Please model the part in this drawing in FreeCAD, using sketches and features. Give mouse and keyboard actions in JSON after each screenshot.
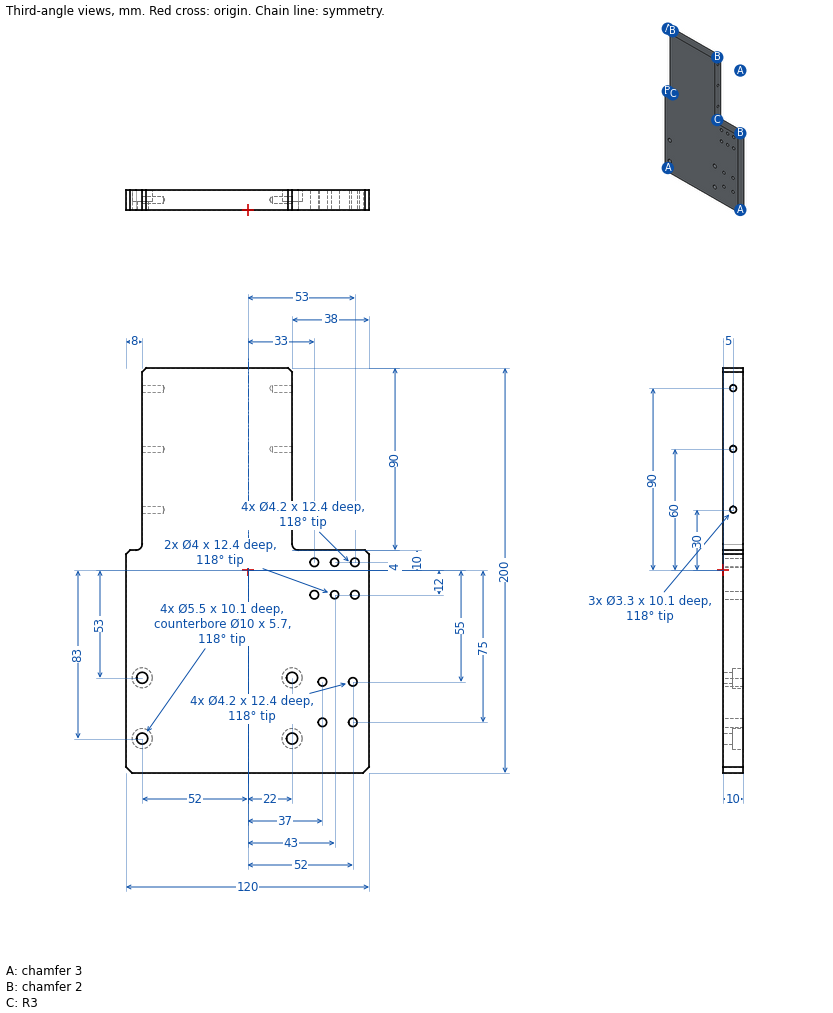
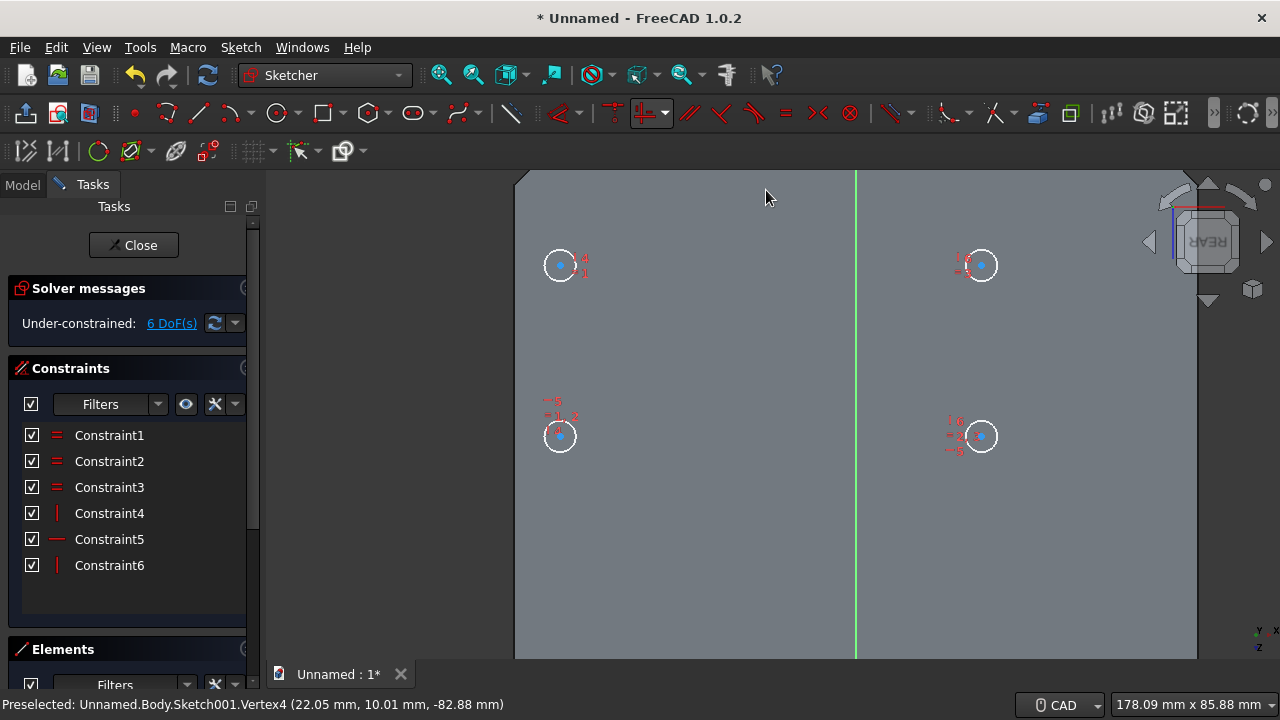
{"action": "left_click", "coordinate": [560, 266]}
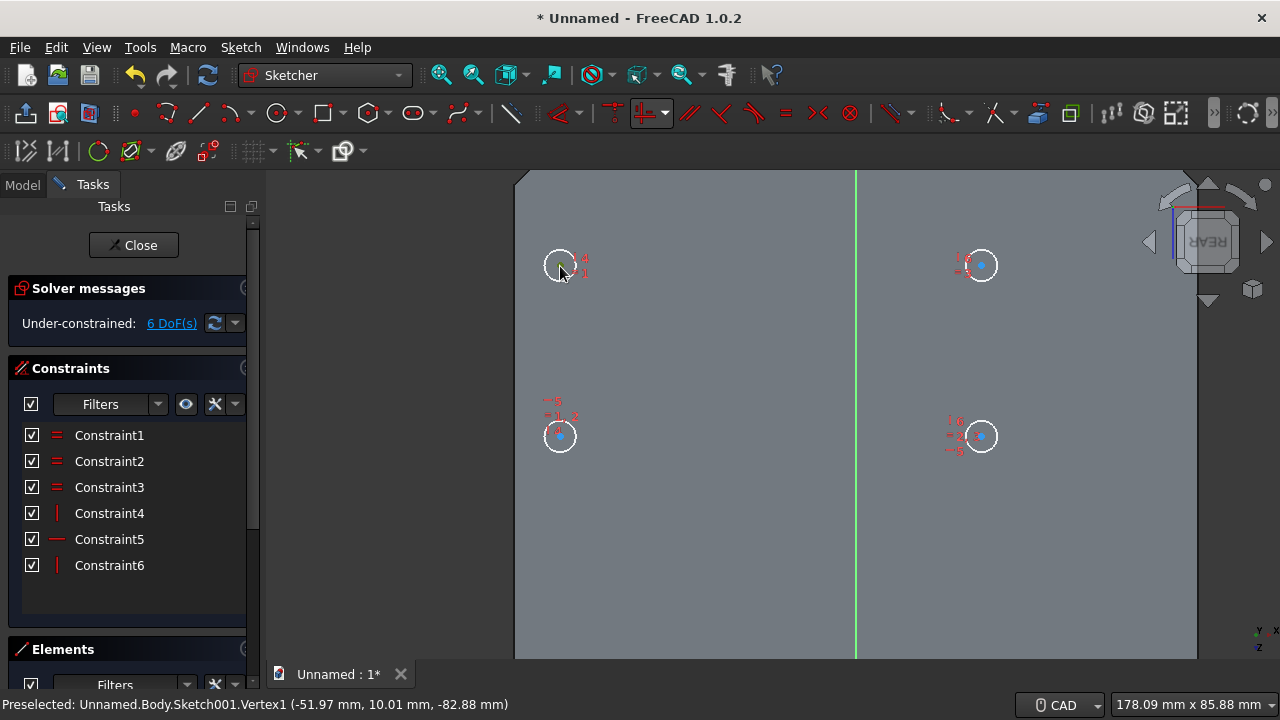
{"action": "left_click", "coordinate": [982, 266]}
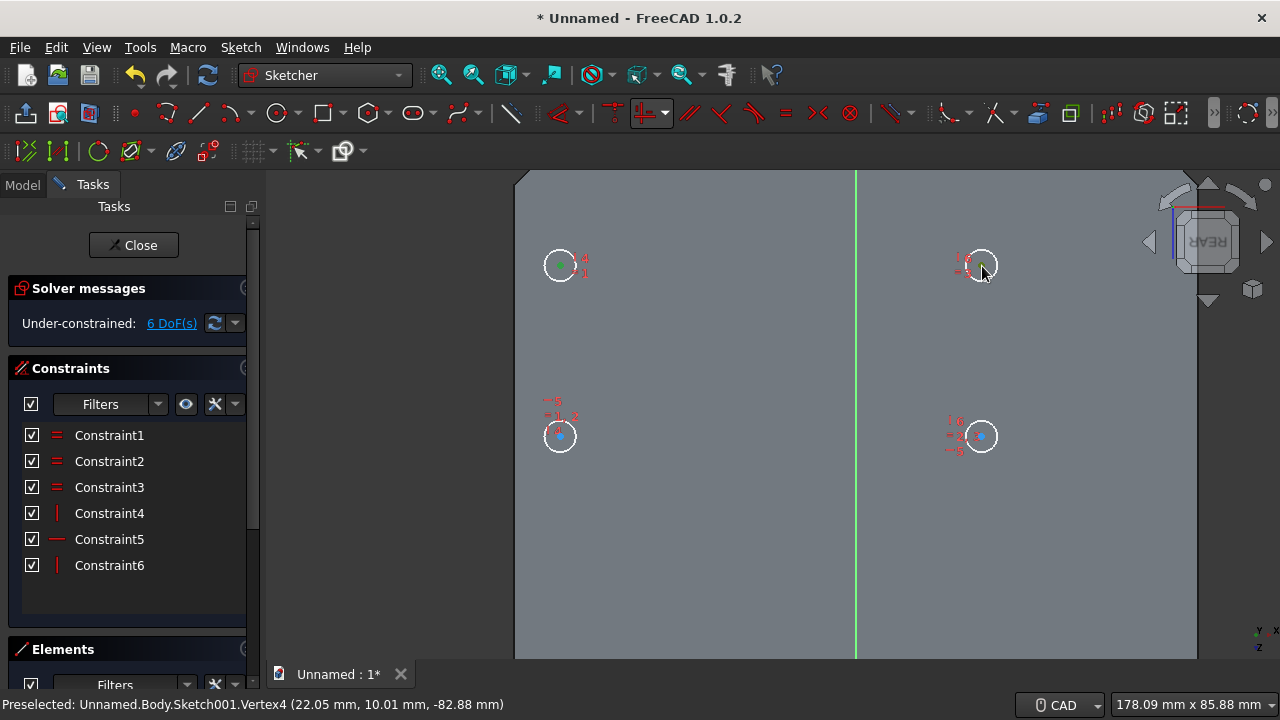
{"action": "key", "text": "h"}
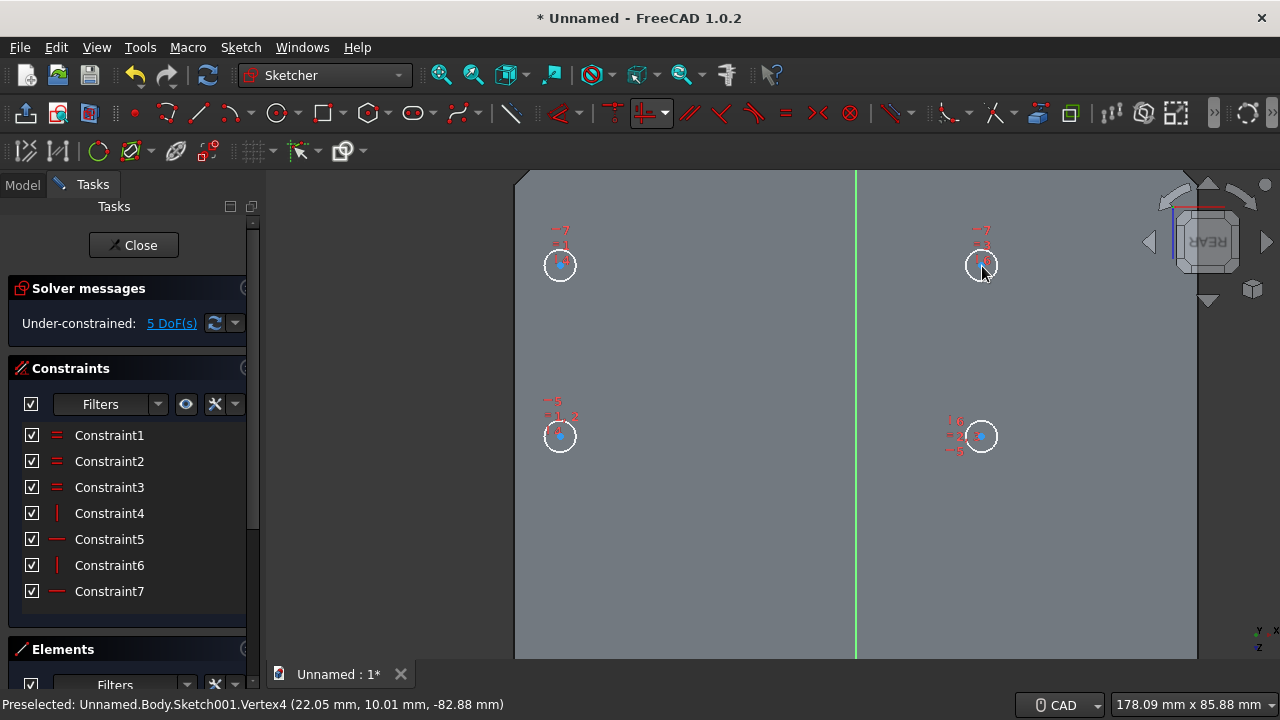
{"action": "left_click", "coordinate": [558, 114]}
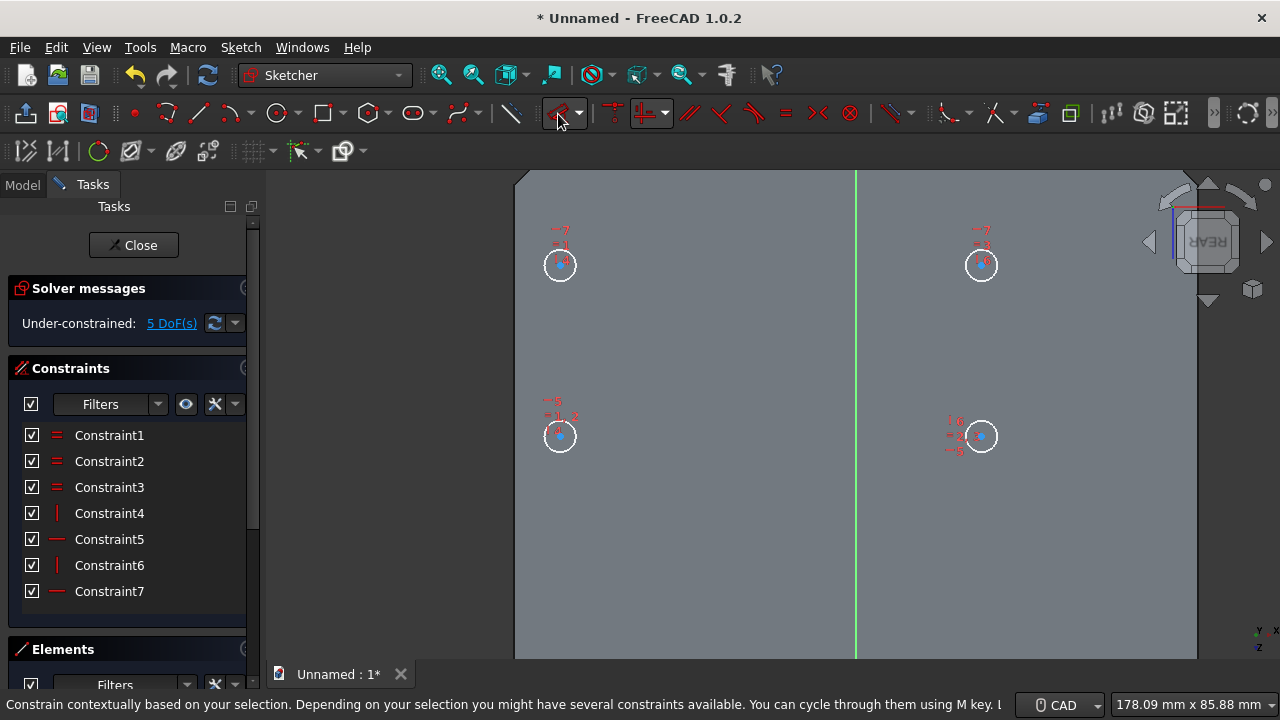
{"action": "scroll", "coordinate": [571, 254], "scroll_direction": "up", "scroll_amount": 2}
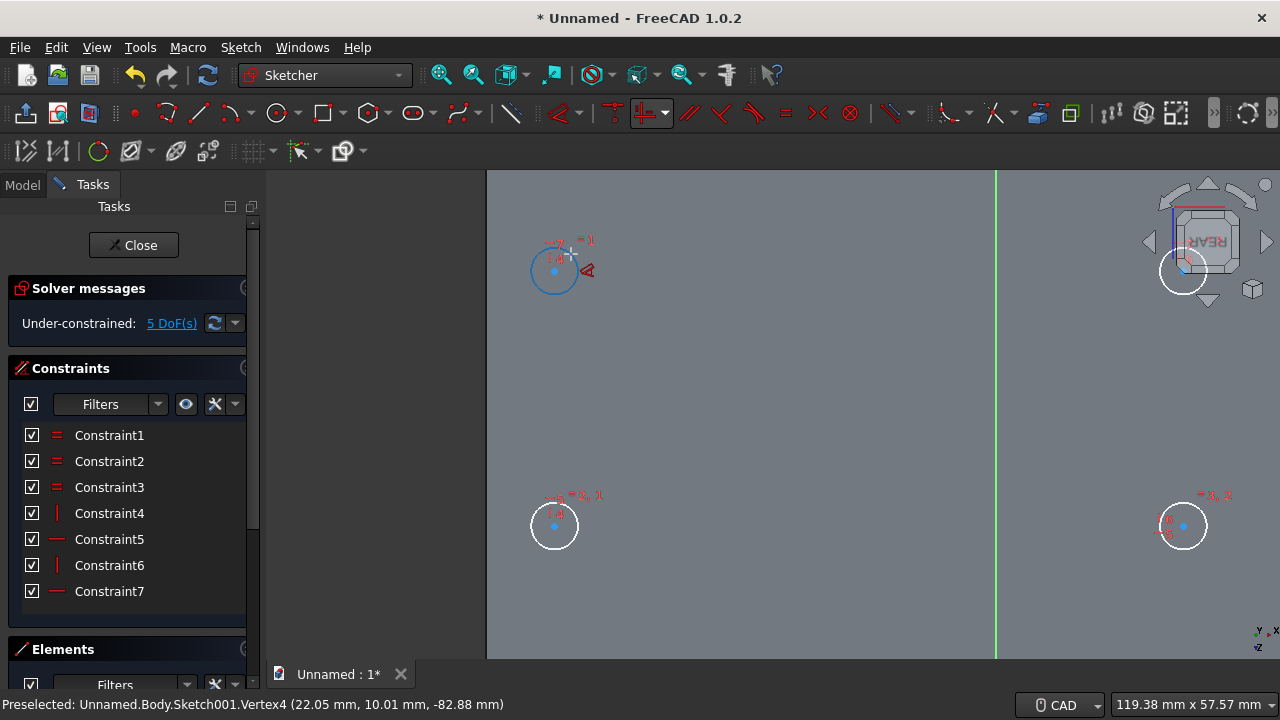
{"action": "left_click", "coordinate": [571, 255]}
{"action": "left_click", "coordinate": [594, 233]}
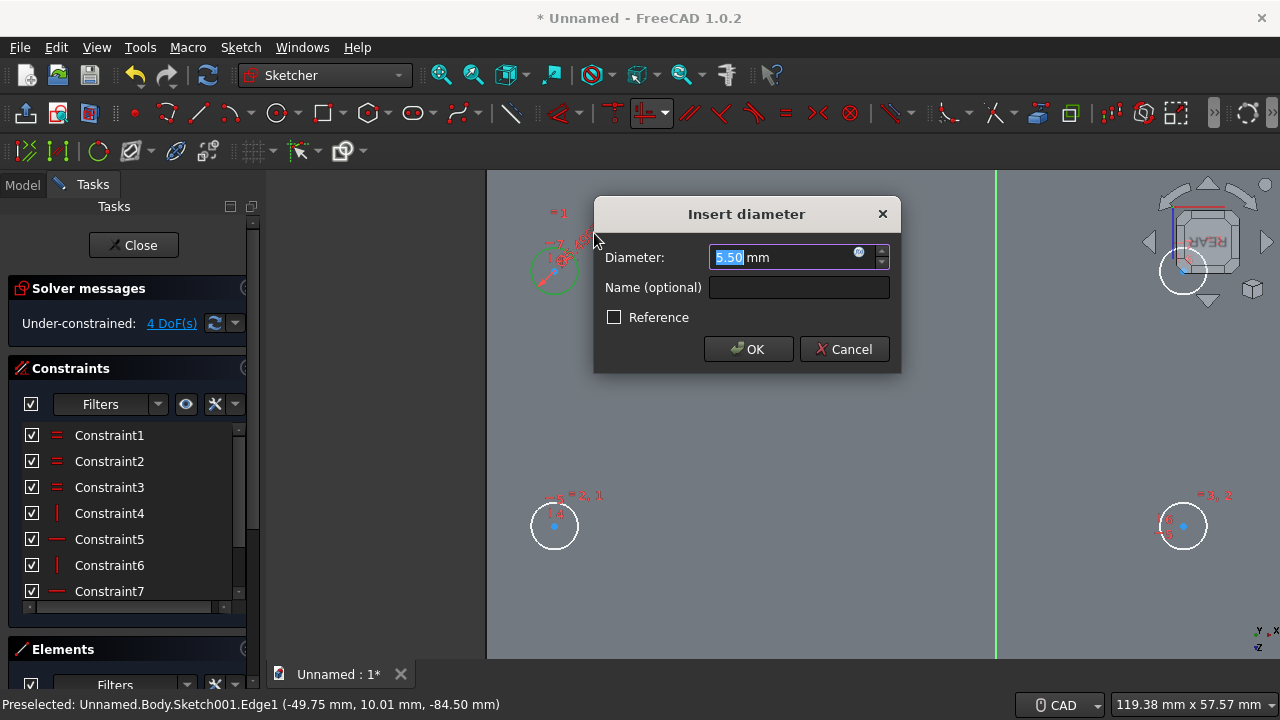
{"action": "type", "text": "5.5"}
{"action": "key", "text": "Return"}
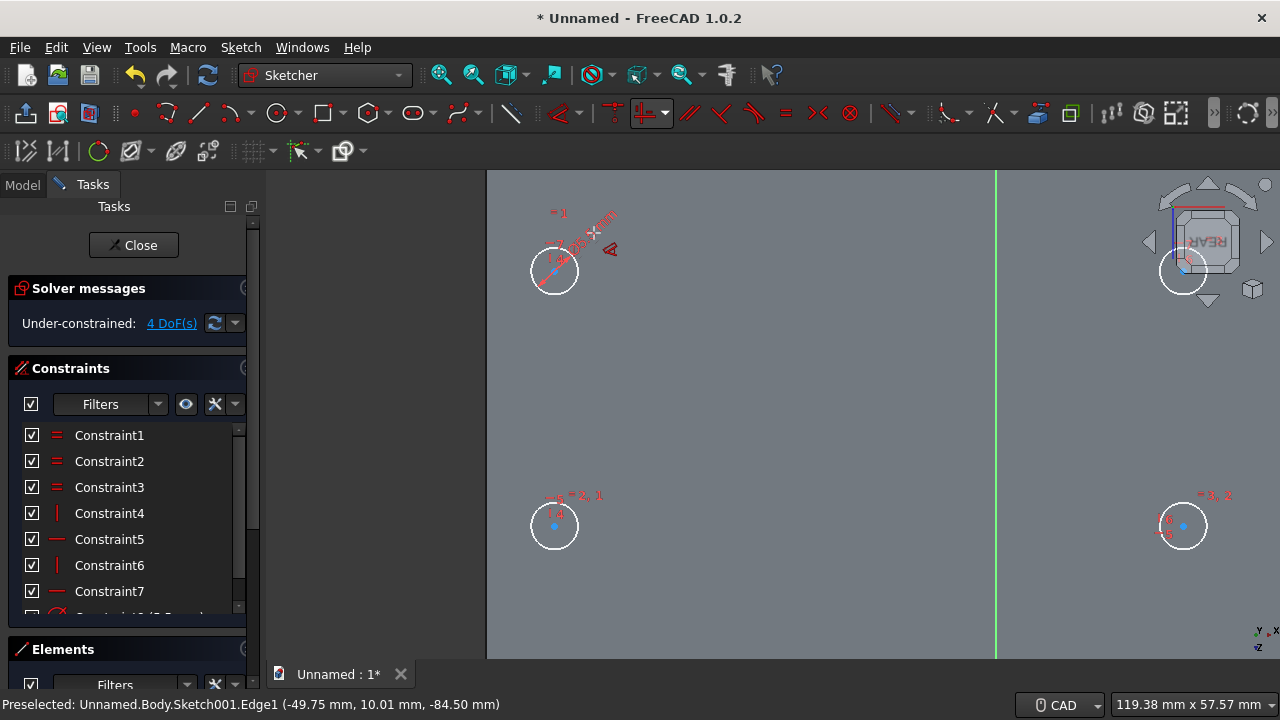
{"action": "left_click", "coordinate": [555, 271]}
{"action": "left_click", "coordinate": [775, 237]}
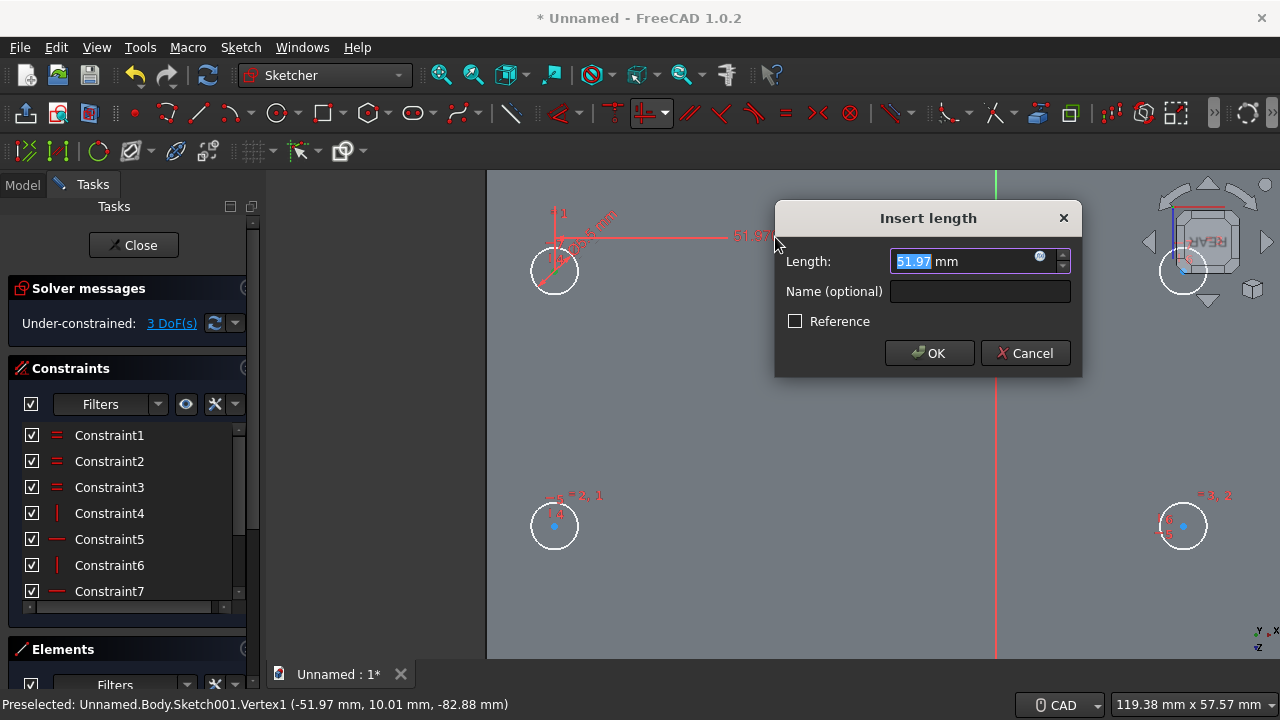
{"action": "type", "text": "52"}
{"action": "key", "text": "Return"}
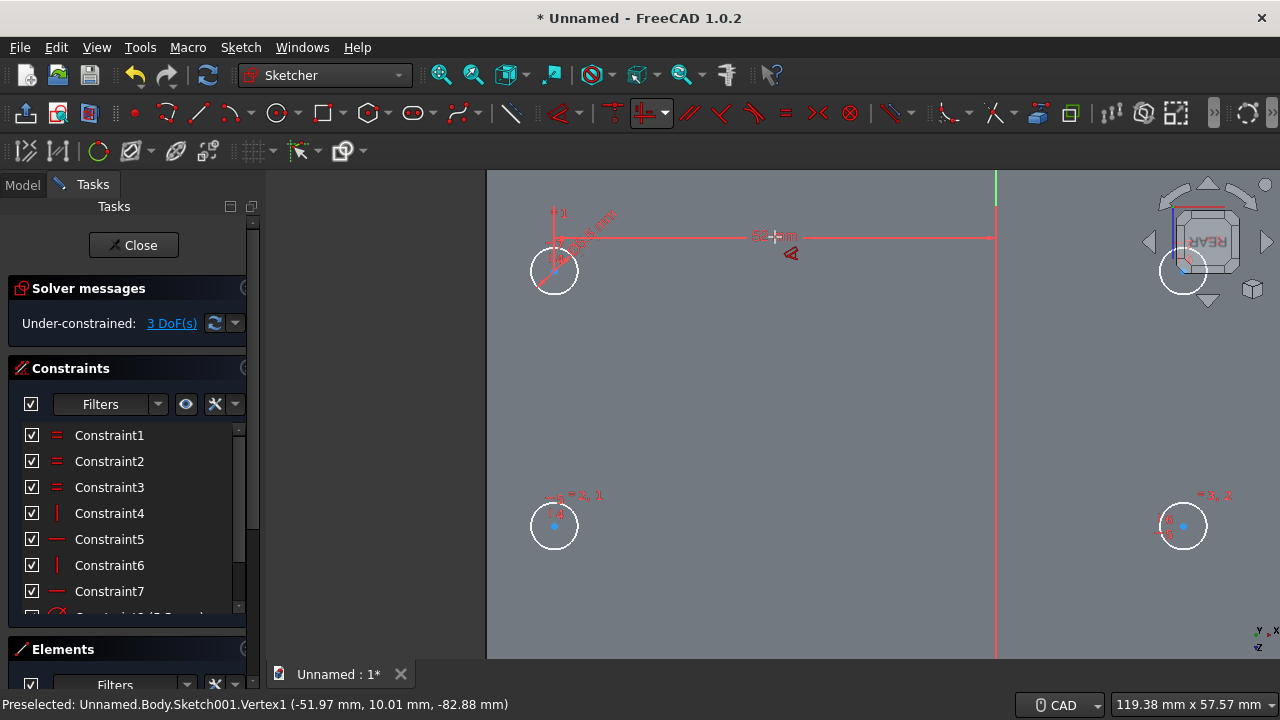
{"action": "left_click", "coordinate": [554, 271]}
{"action": "left_click", "coordinate": [520, 451]}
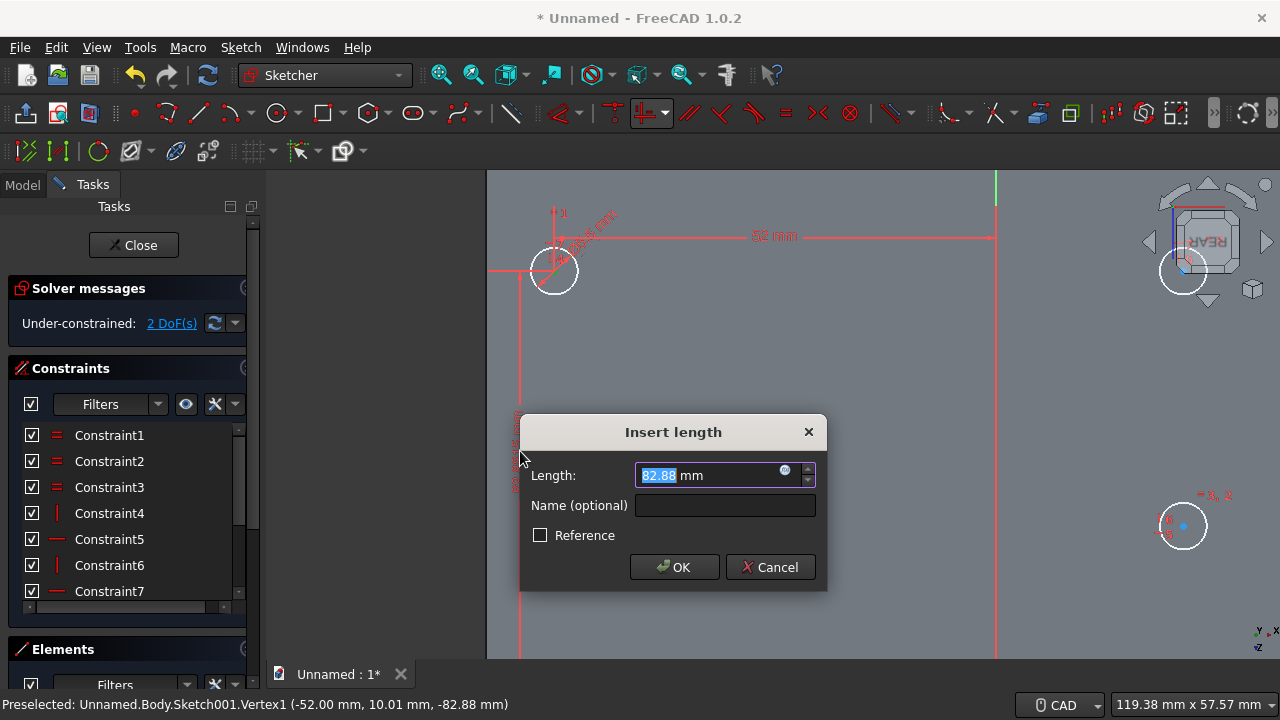
{"action": "type", "text": "83"}
{"action": "key", "text": "Return"}